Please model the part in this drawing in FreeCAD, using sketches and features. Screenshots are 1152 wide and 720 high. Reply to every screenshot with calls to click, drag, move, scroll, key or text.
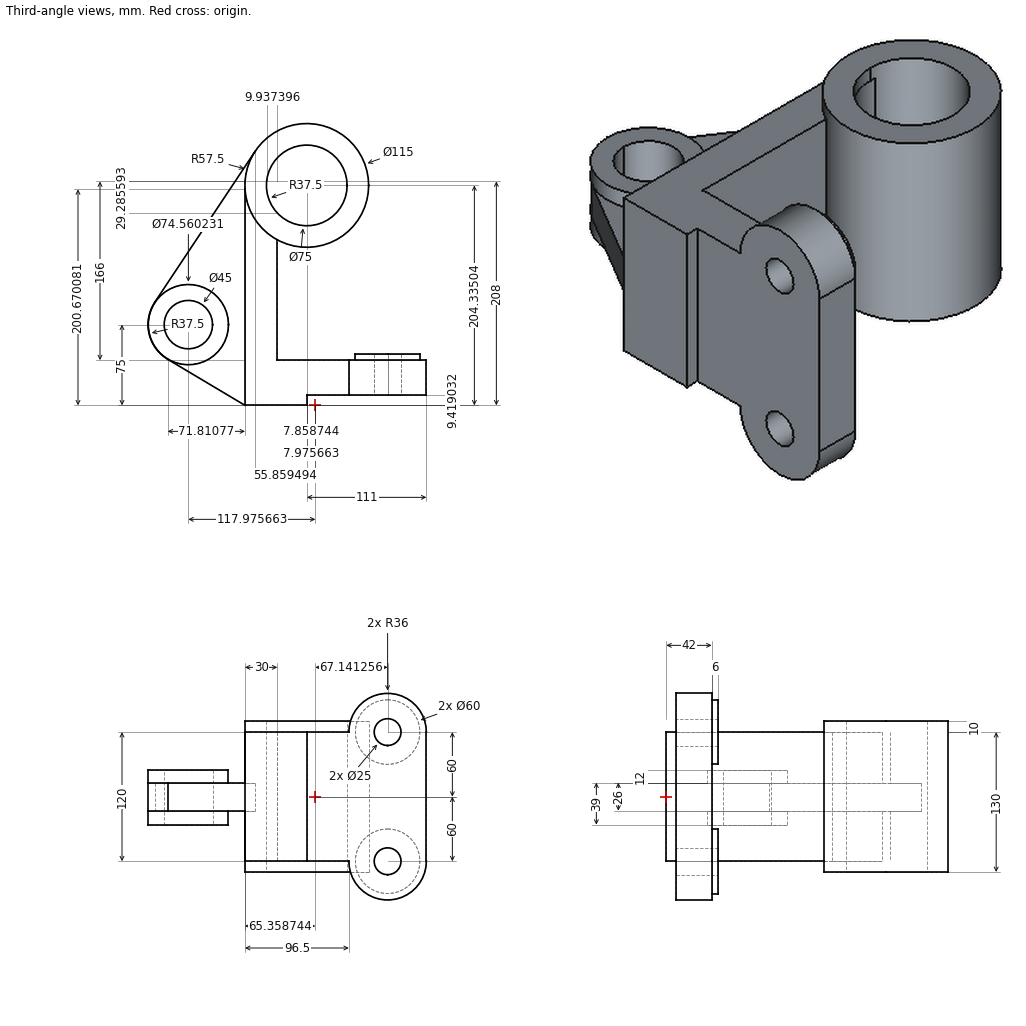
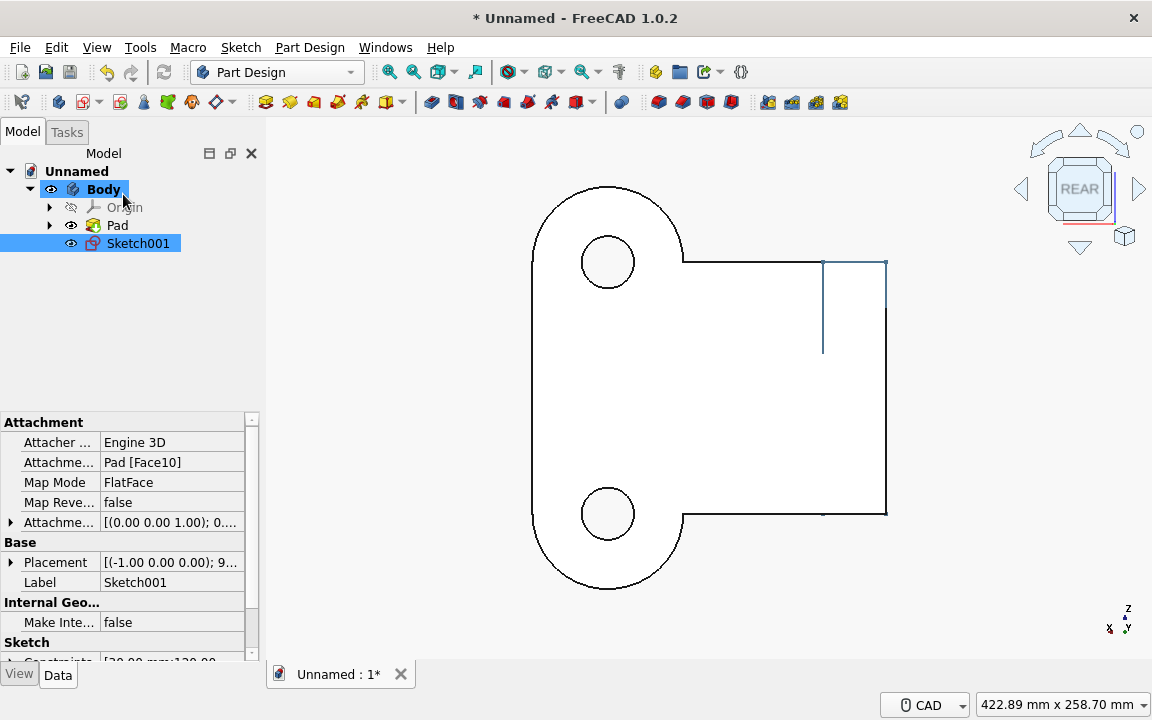
click(266, 102)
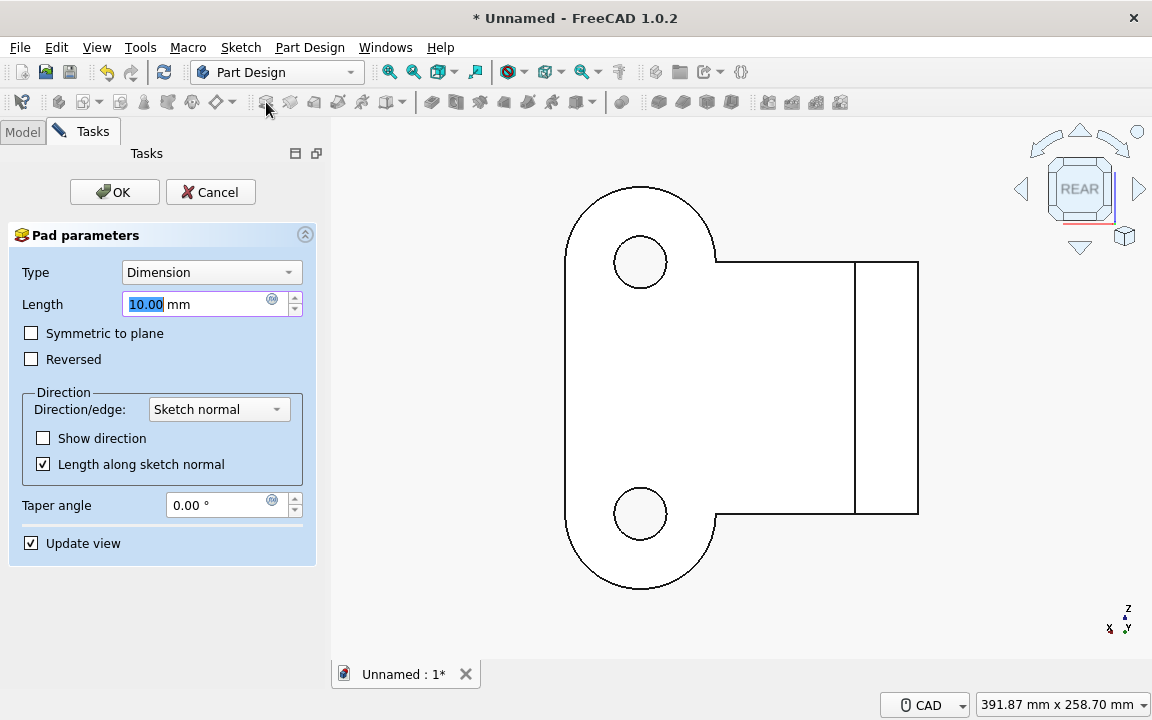
text(166)
key(Tab)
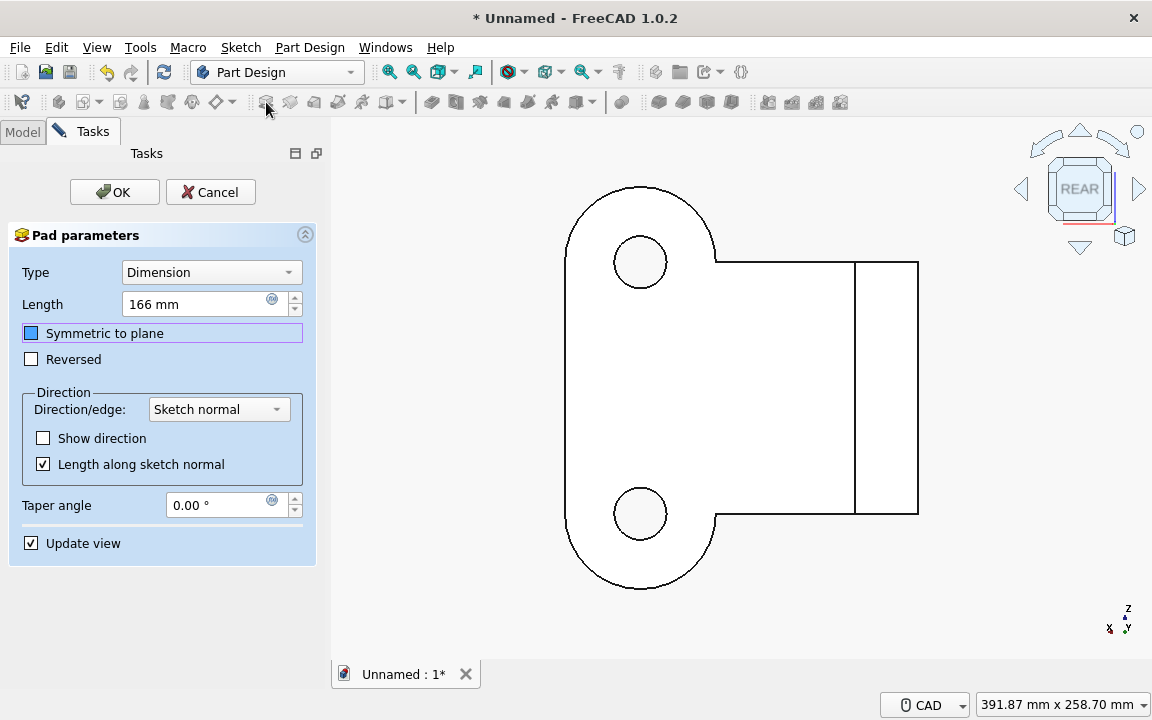
click(115, 192)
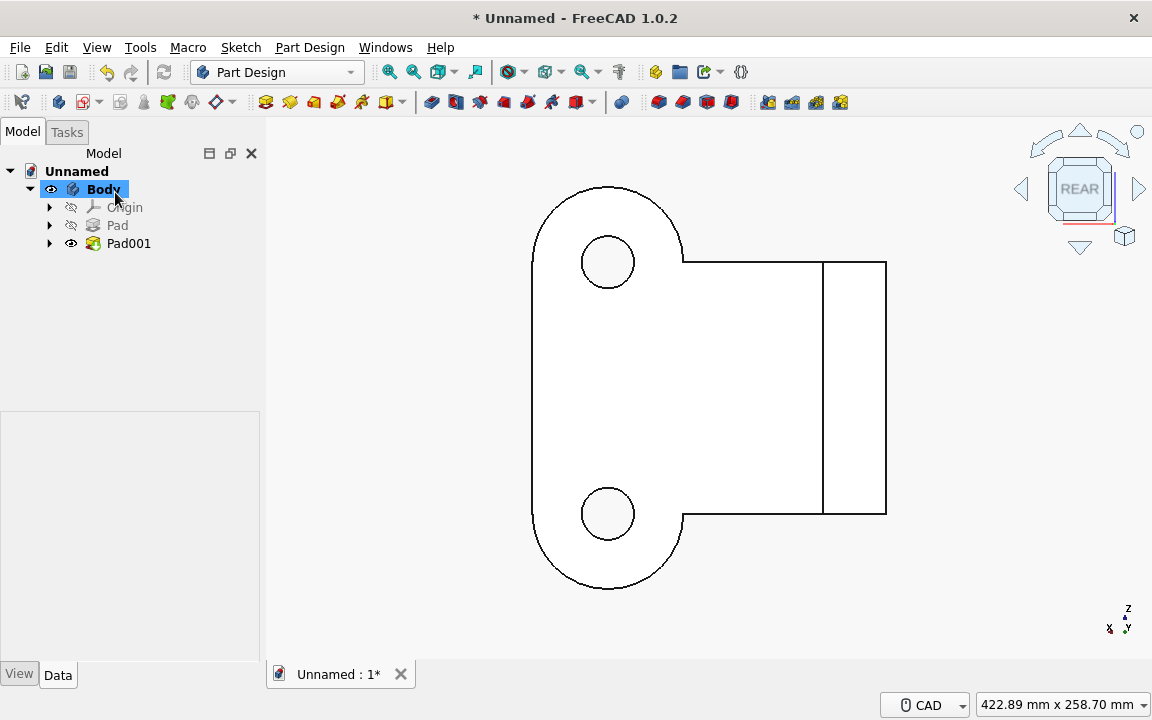
key(0)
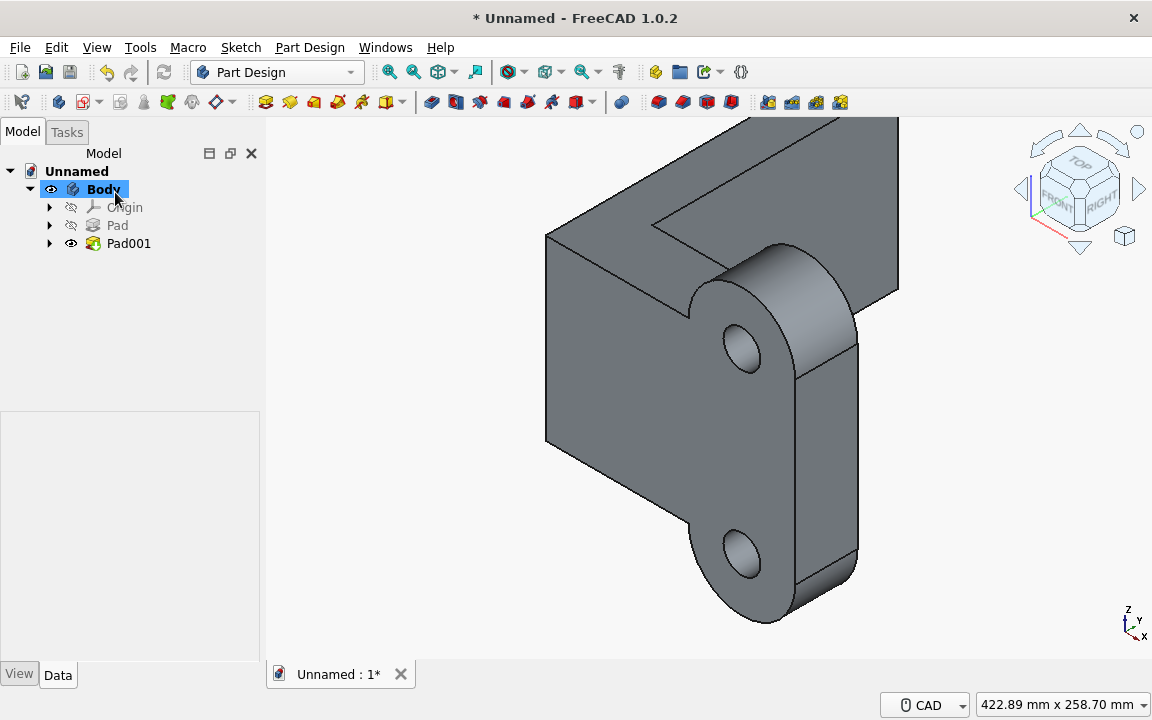
click(390, 72)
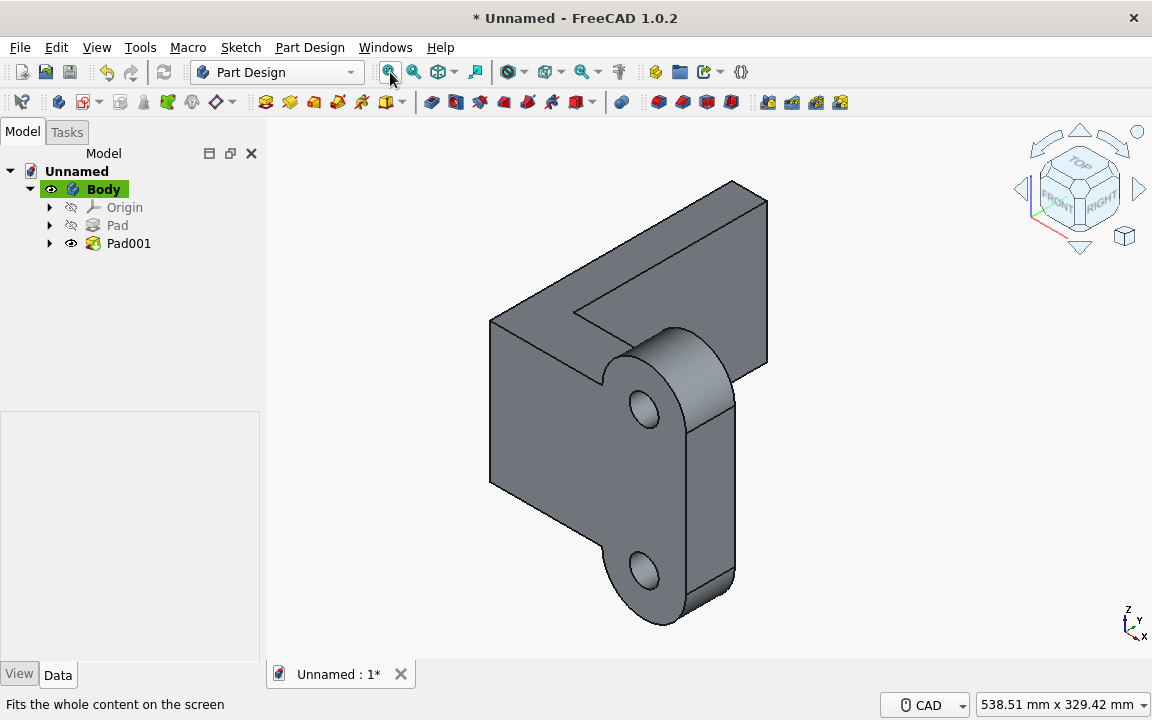
click(595, 361)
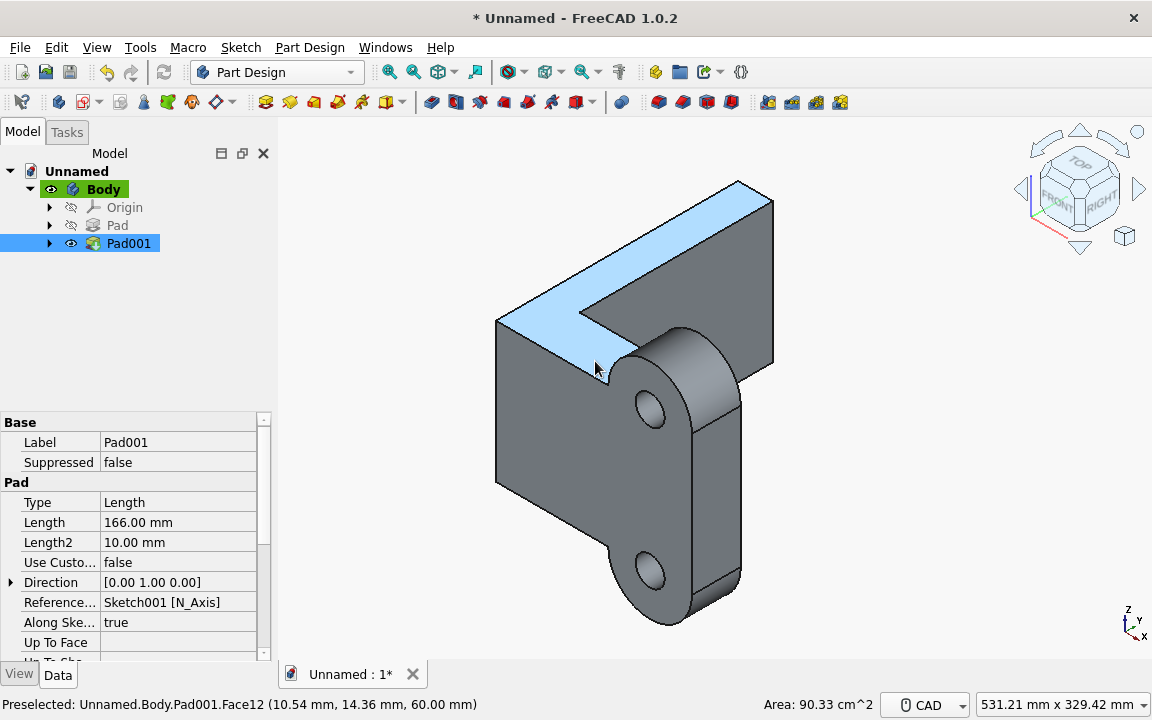
click(84, 102)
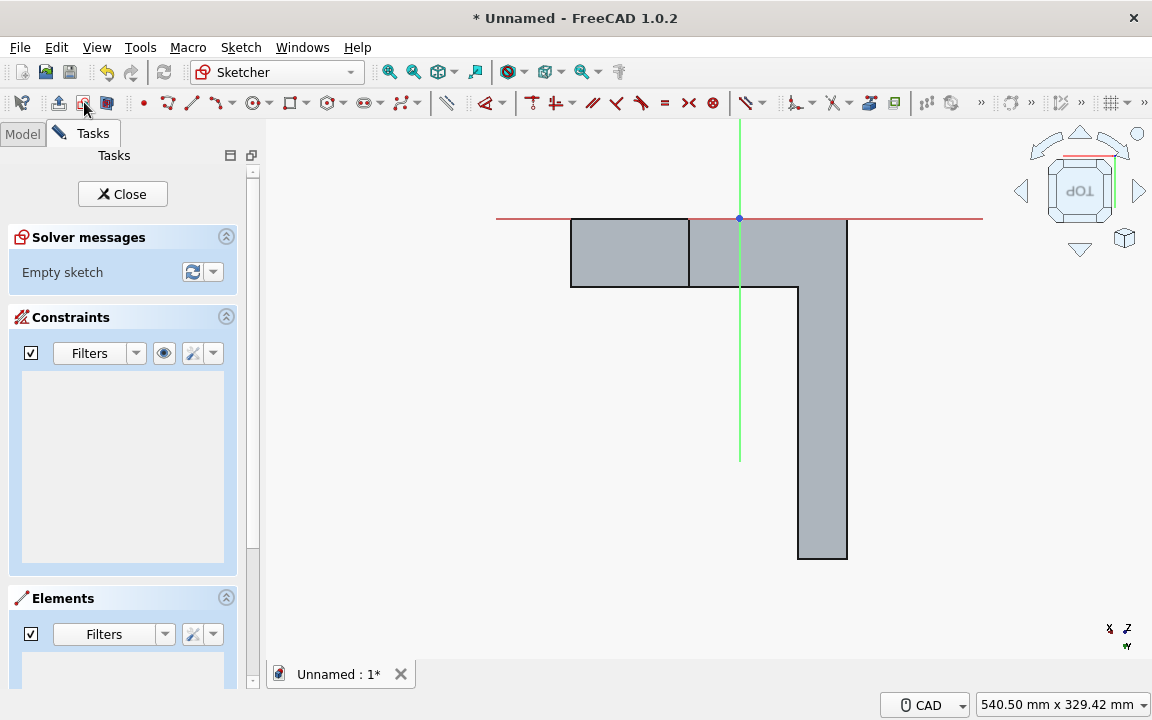
click(108, 104)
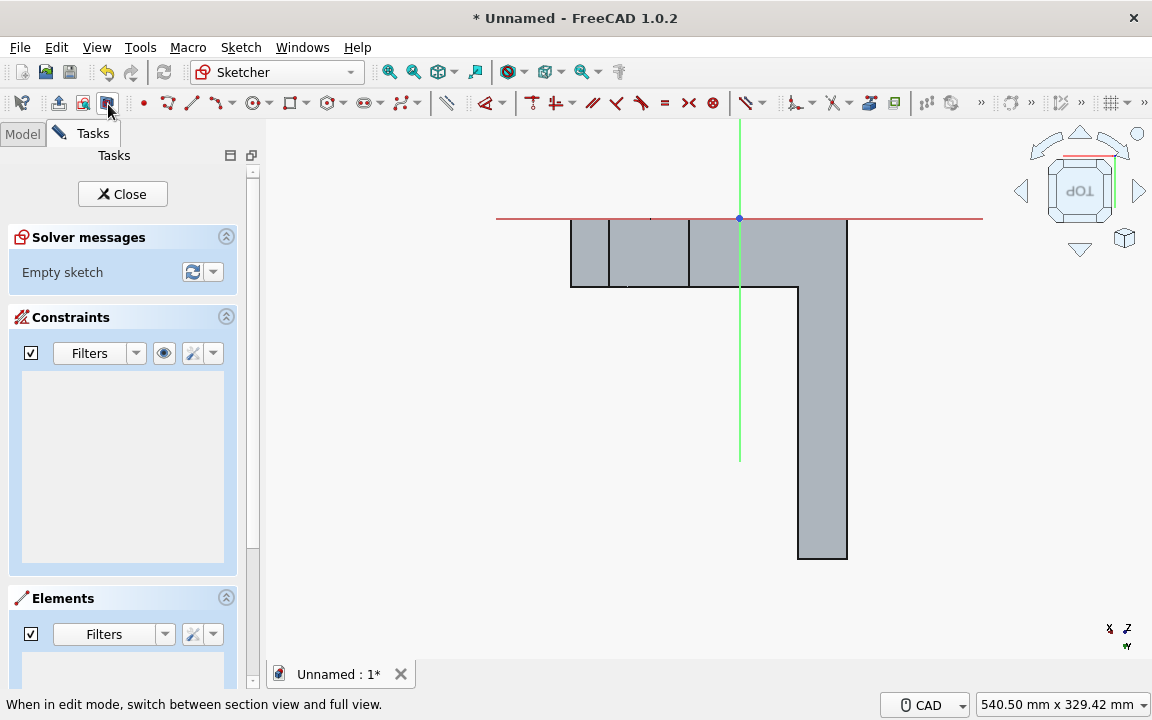
scroll(294, 190, down, 1)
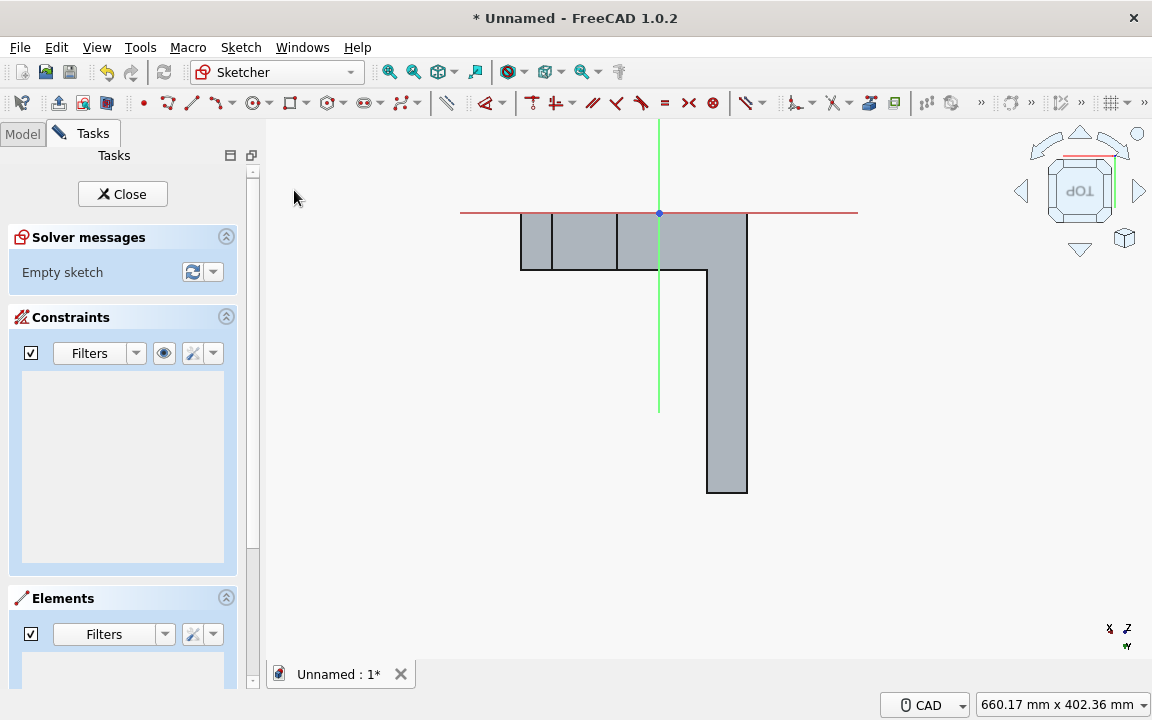
click(254, 104)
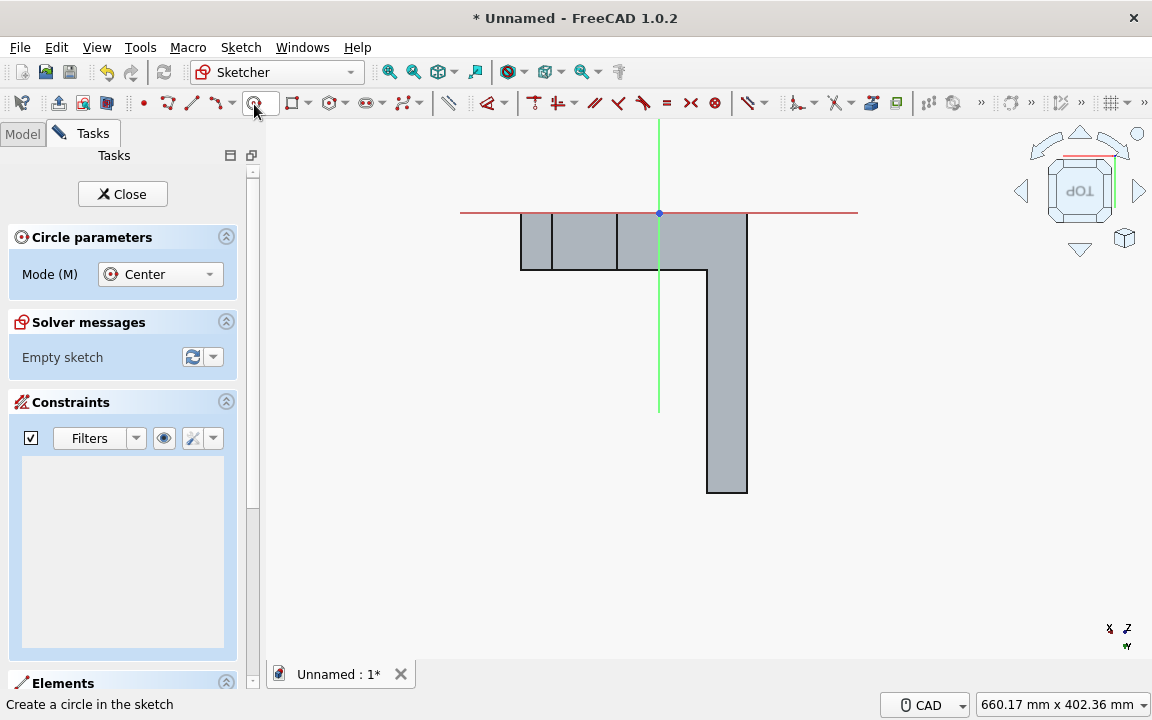
scroll(670, 488, up, 2)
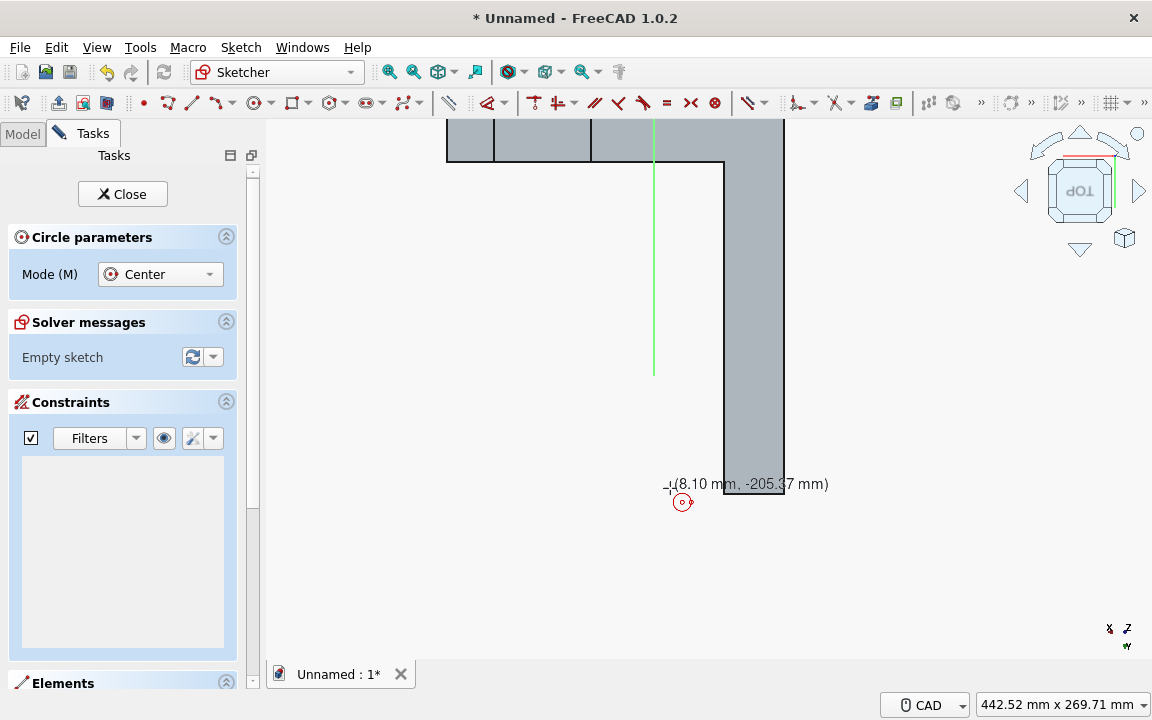
click(670, 487)
move(751, 406)